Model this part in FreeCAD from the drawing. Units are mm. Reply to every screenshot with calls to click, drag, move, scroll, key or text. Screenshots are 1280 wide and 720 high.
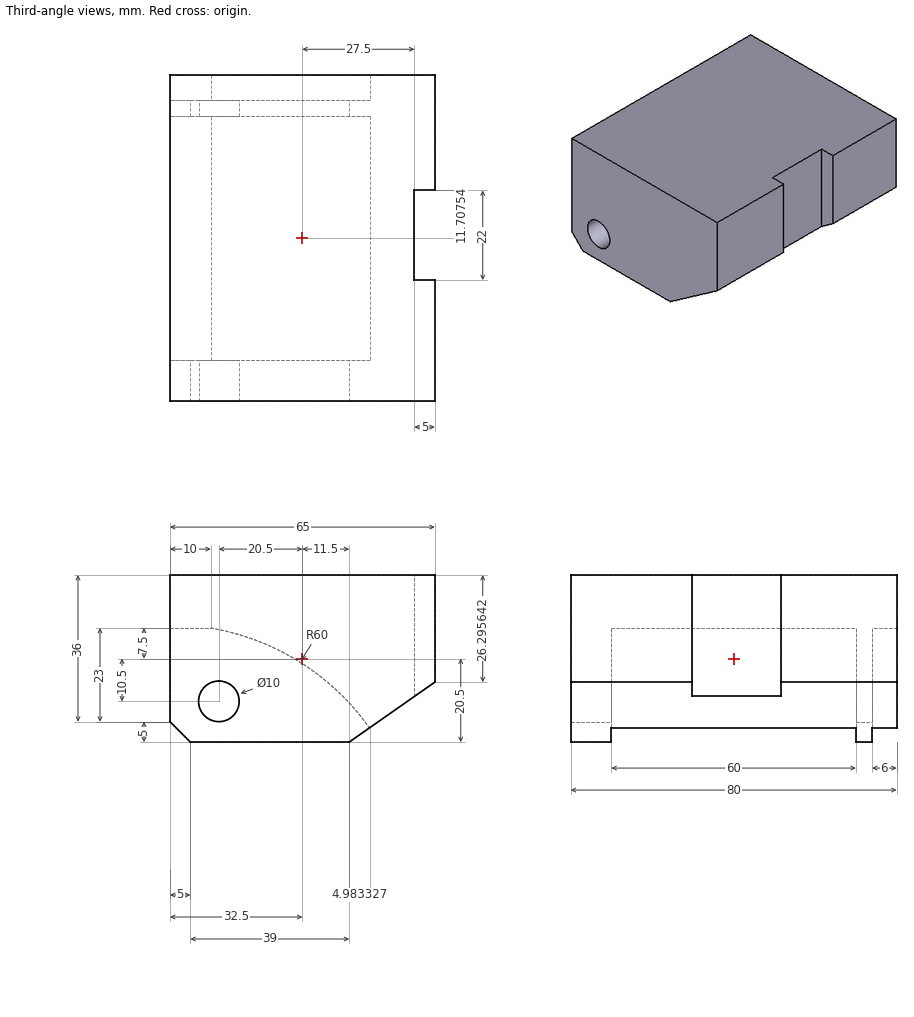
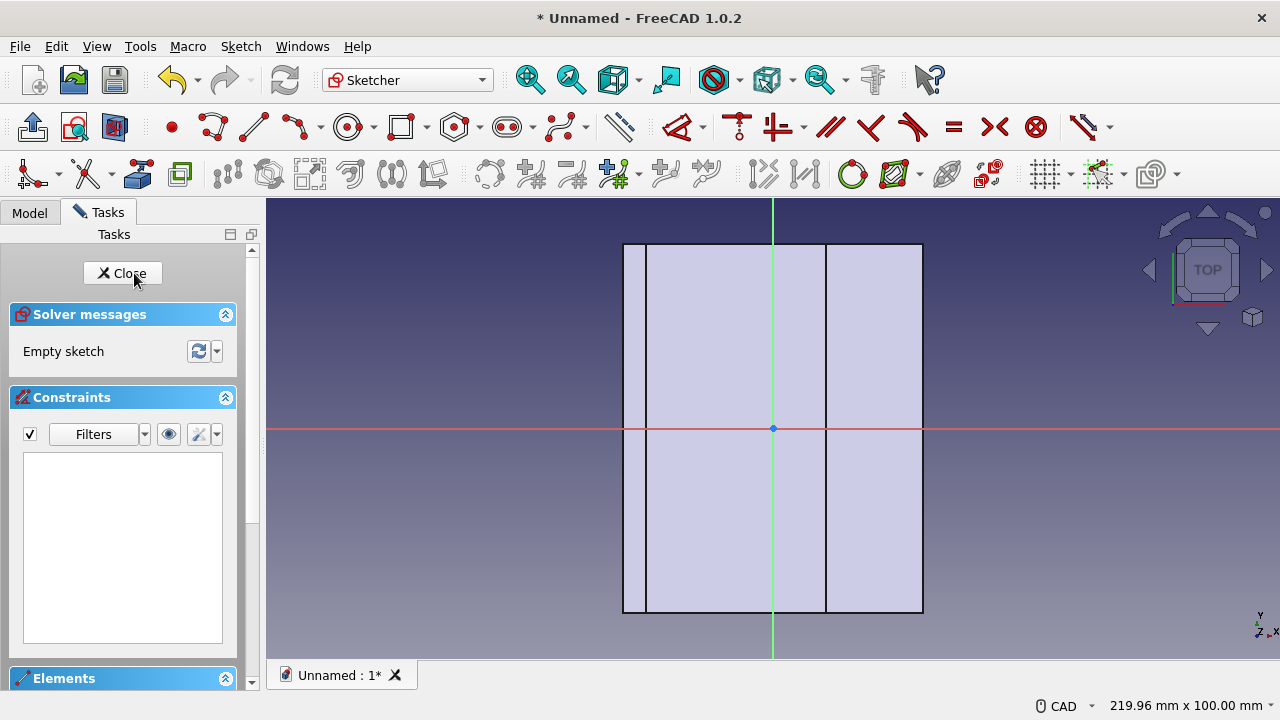
scroll(931, 423, up, 5)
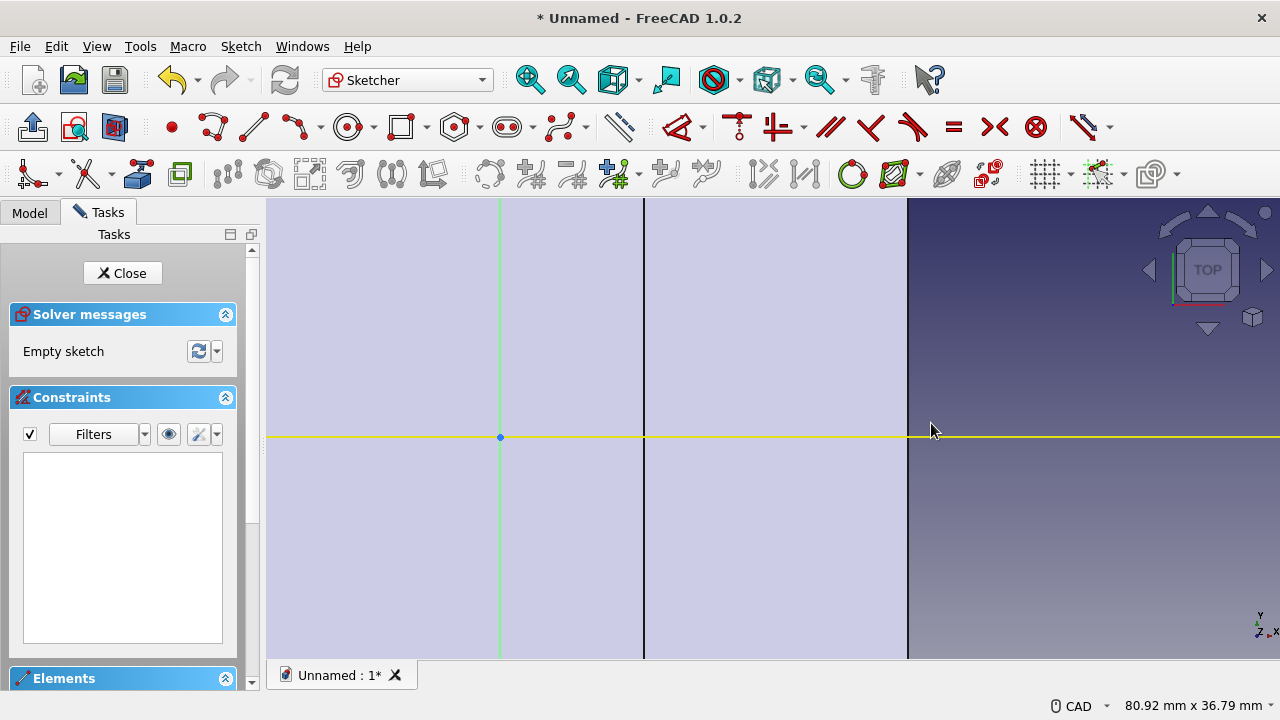
key(g)
key(r)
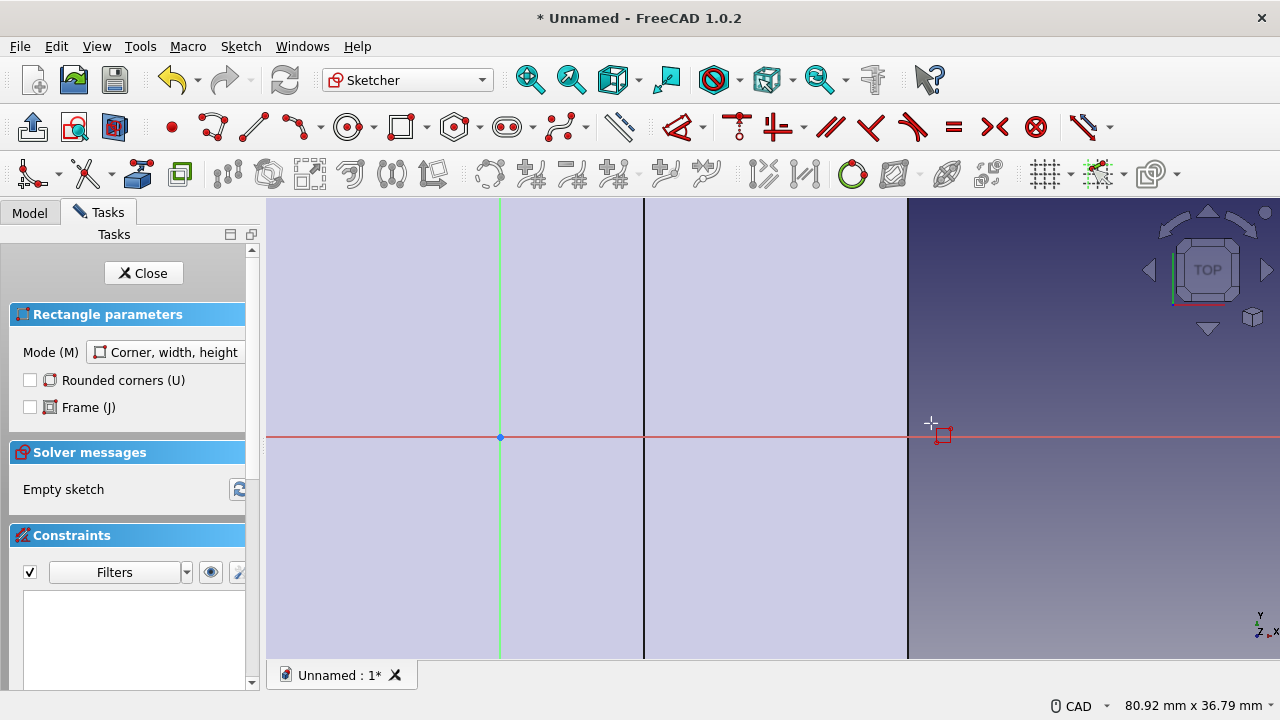
click(845, 290)
click(908, 566)
key(Escape)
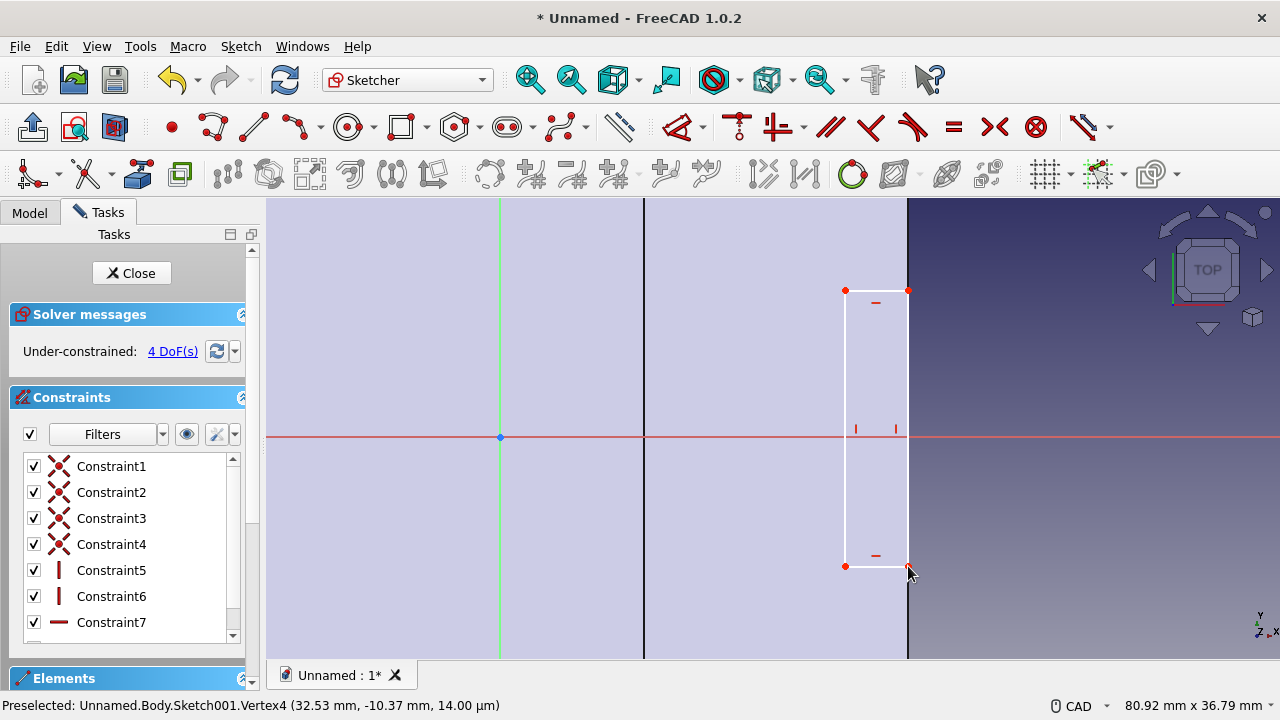
key(d)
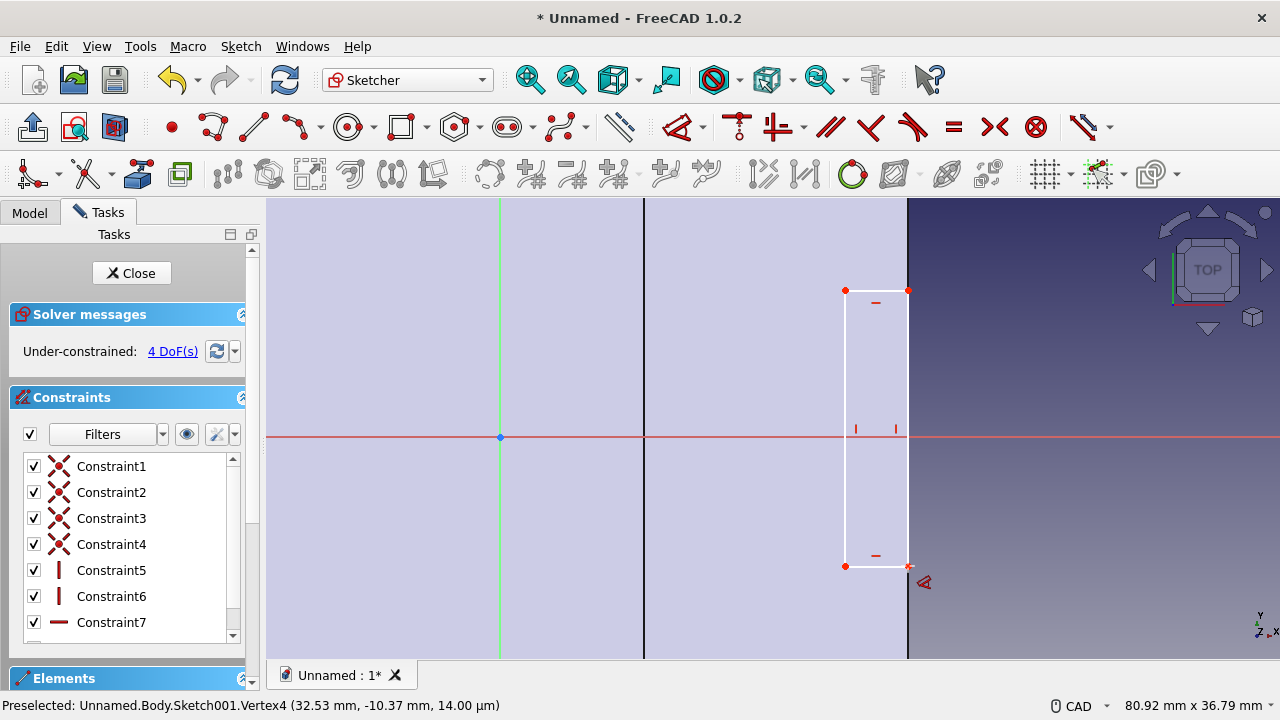
click(864, 567)
click(877, 601)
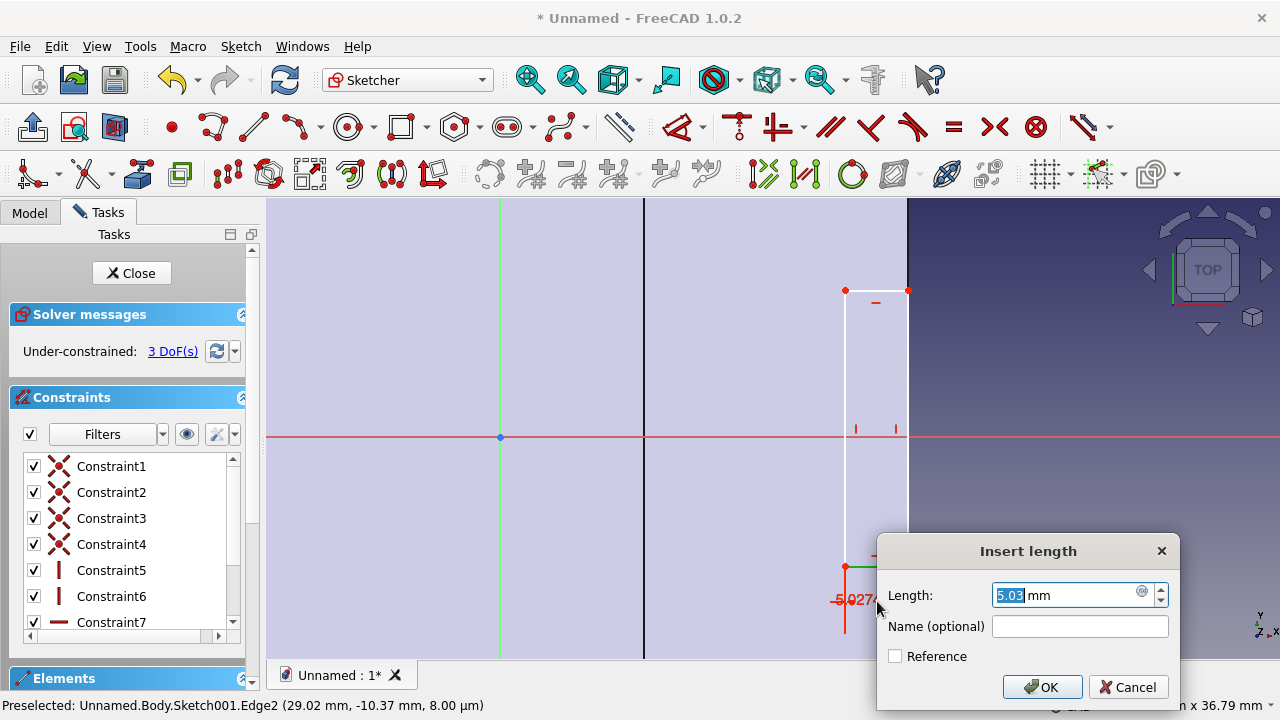
text(5)
key(Return)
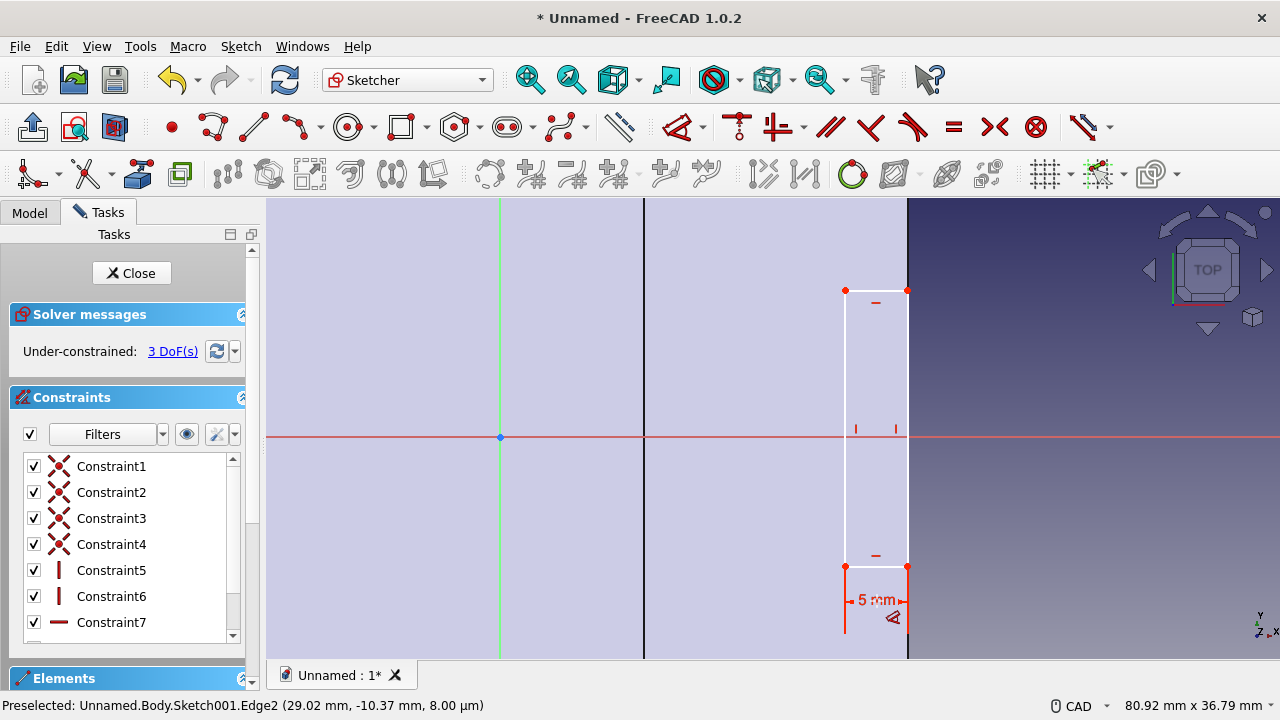
click(845, 374)
click(879, 366)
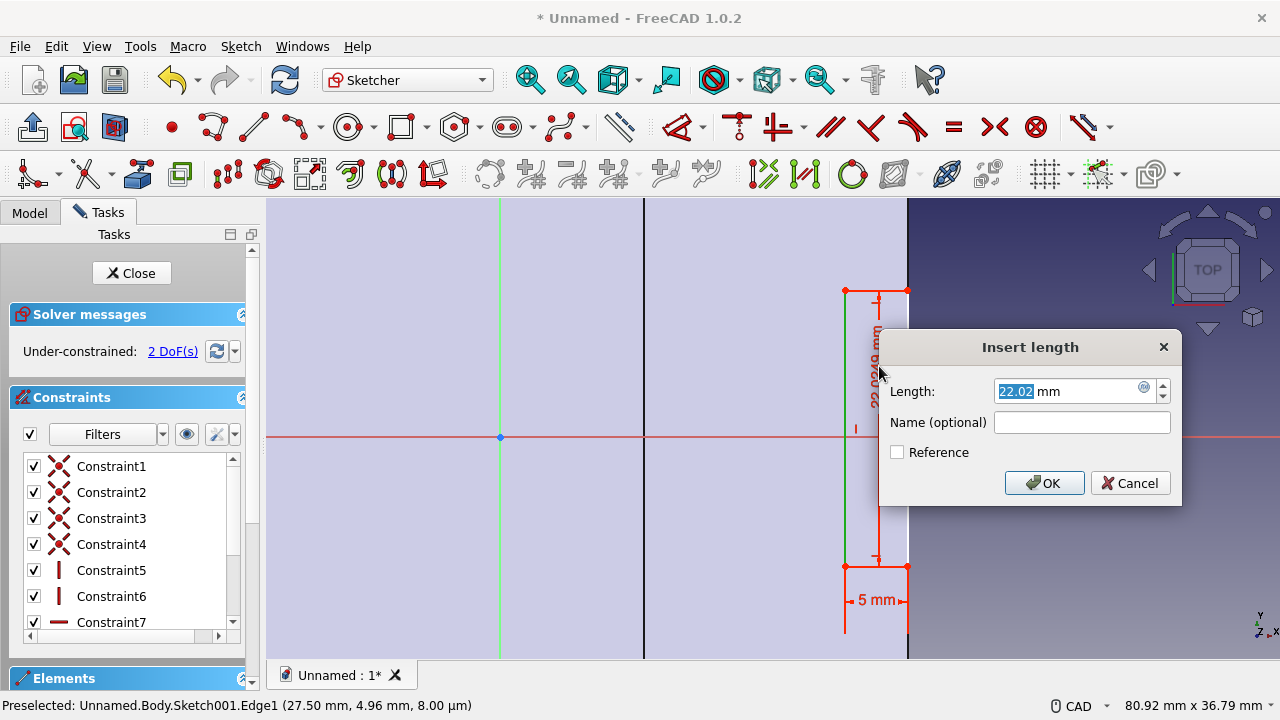
text(22)
key(Return)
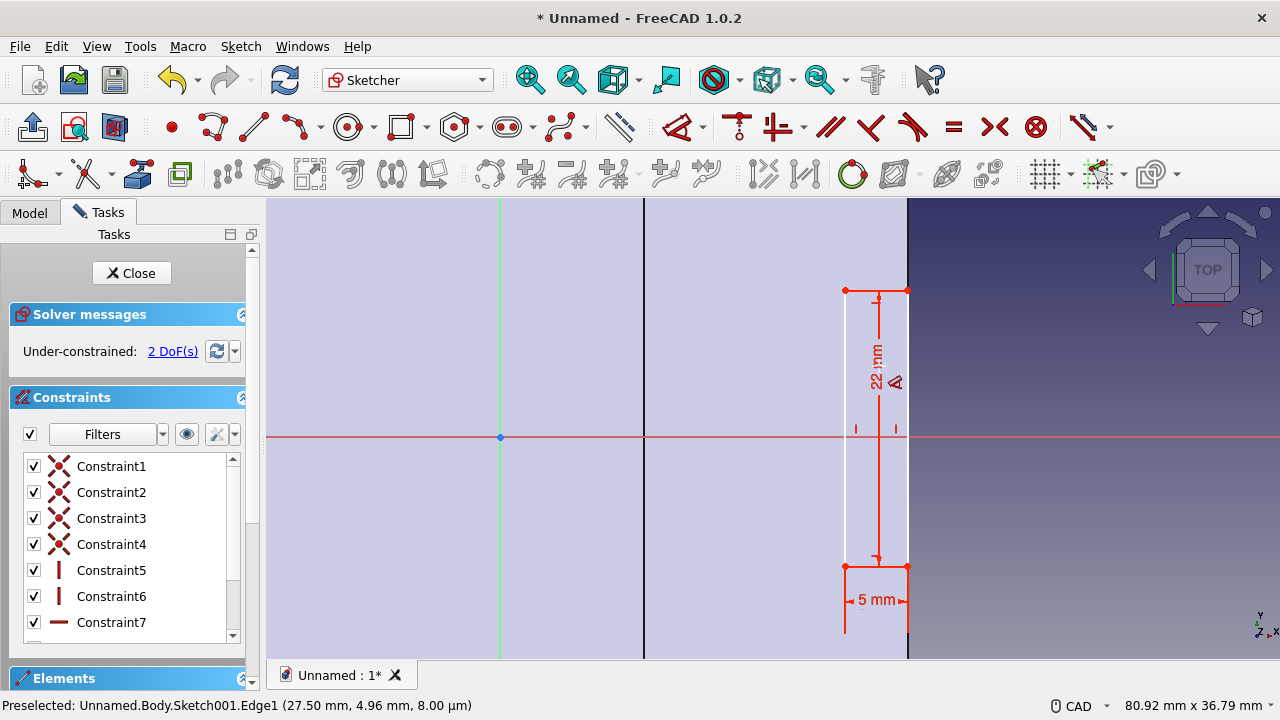
click(845, 291)
click(673, 257)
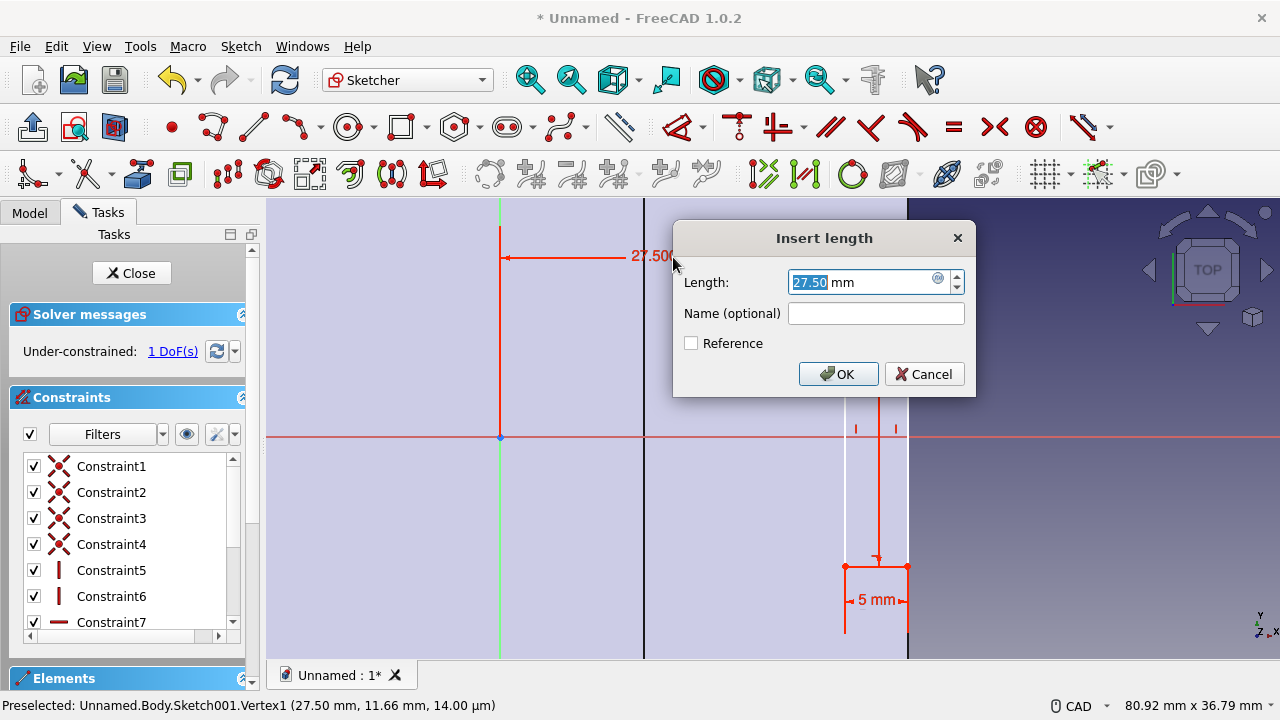
text(27.5)
key(Return)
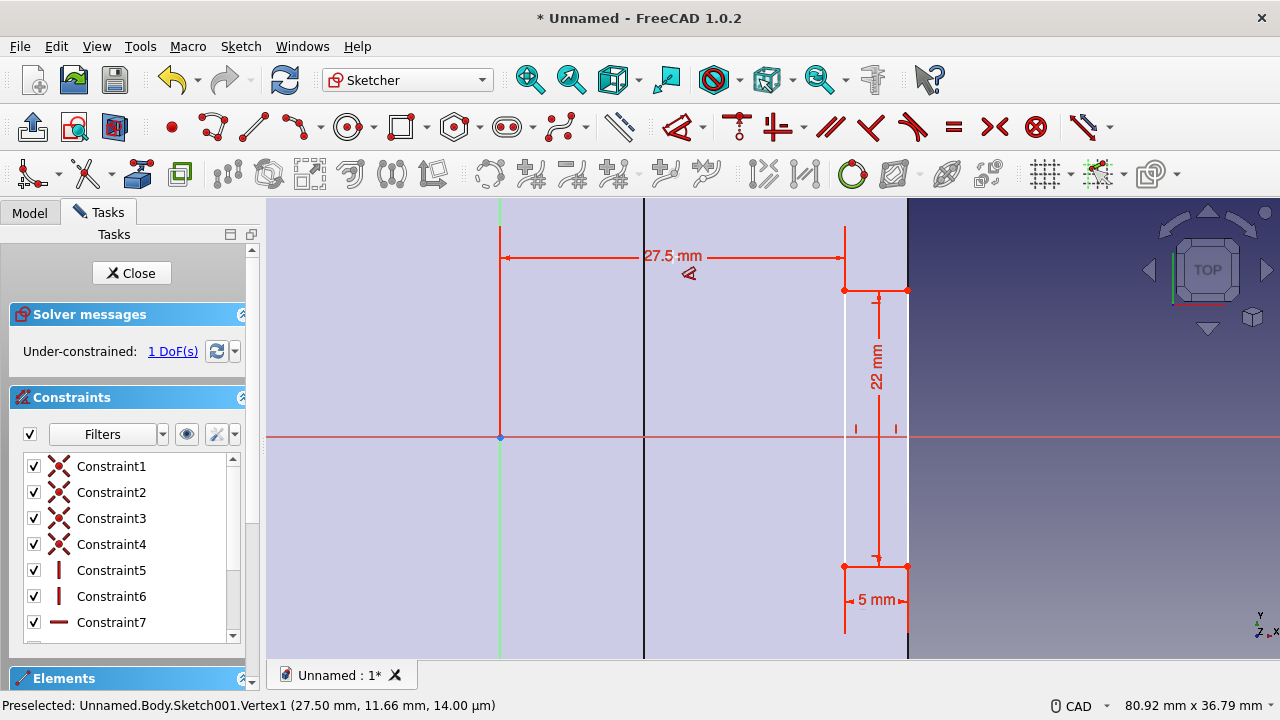
click(845, 291)
click(466, 364)